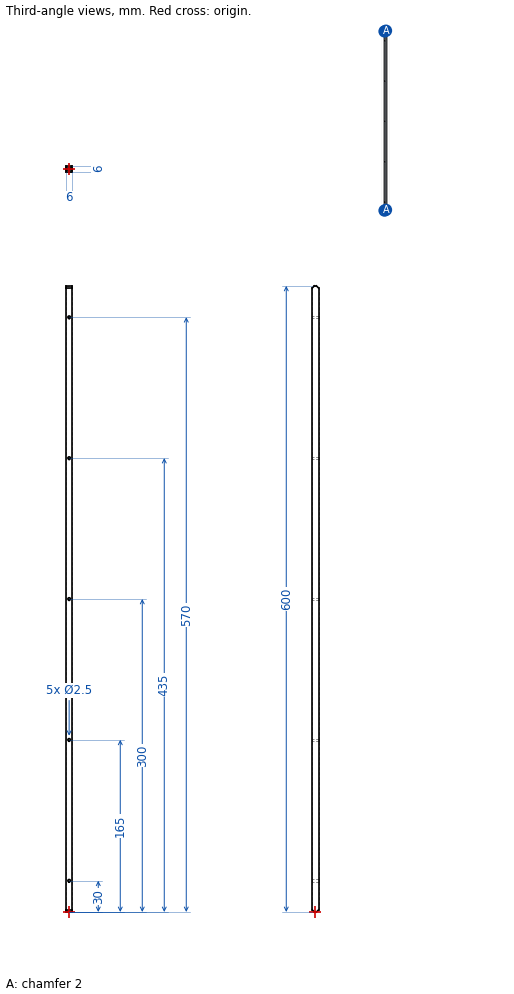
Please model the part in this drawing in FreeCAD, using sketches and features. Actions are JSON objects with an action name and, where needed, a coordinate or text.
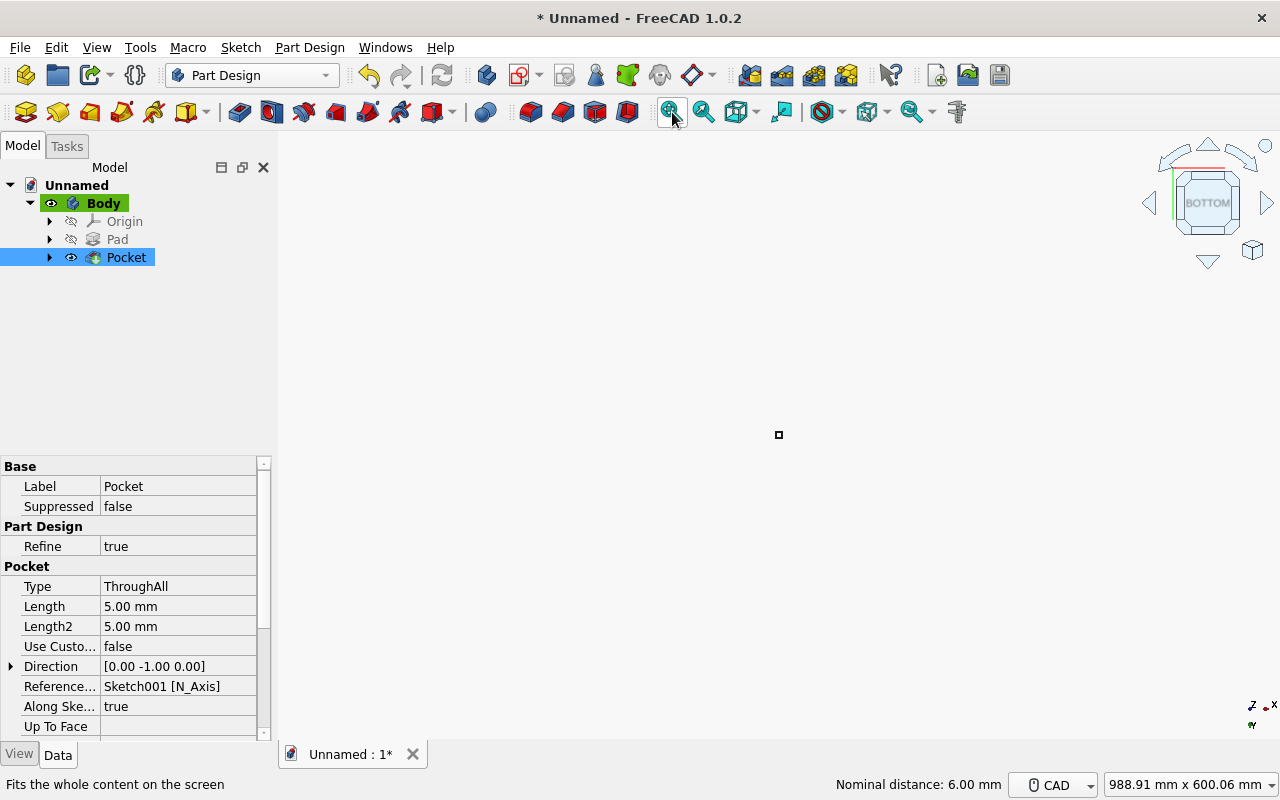
{"action": "scroll", "coordinate": [779, 431], "scroll_direction": "up", "scroll_amount": 10}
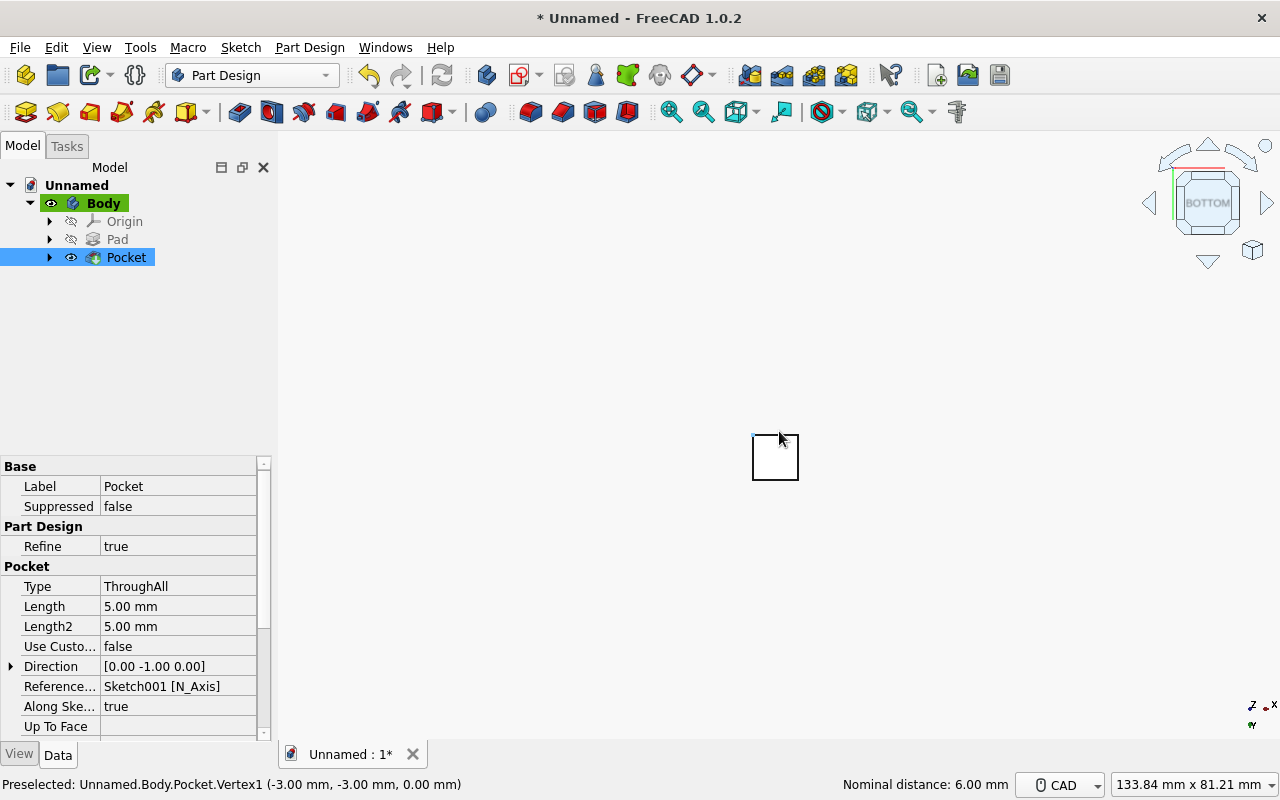
{"action": "left_click", "coordinate": [776, 434], "text": "ctrl"}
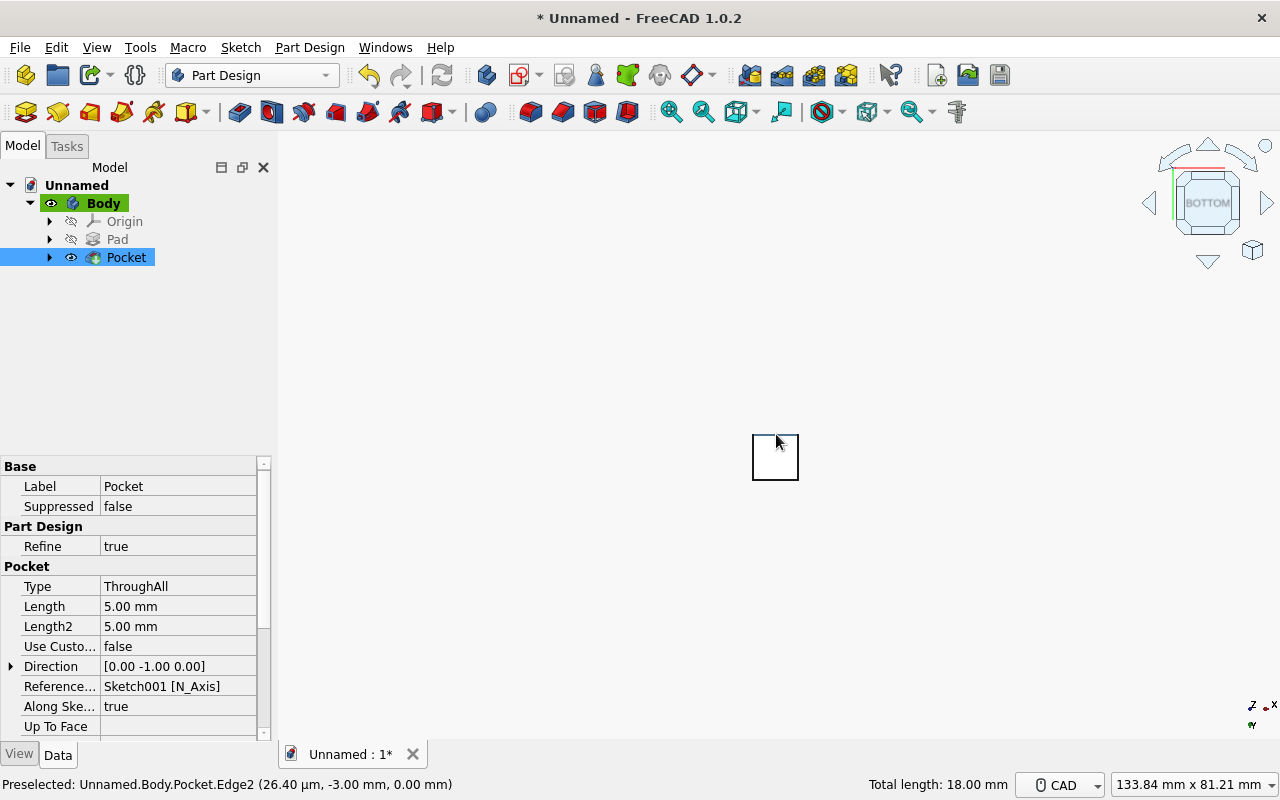
{"action": "left_click", "coordinate": [776, 479], "text": "ctrl"}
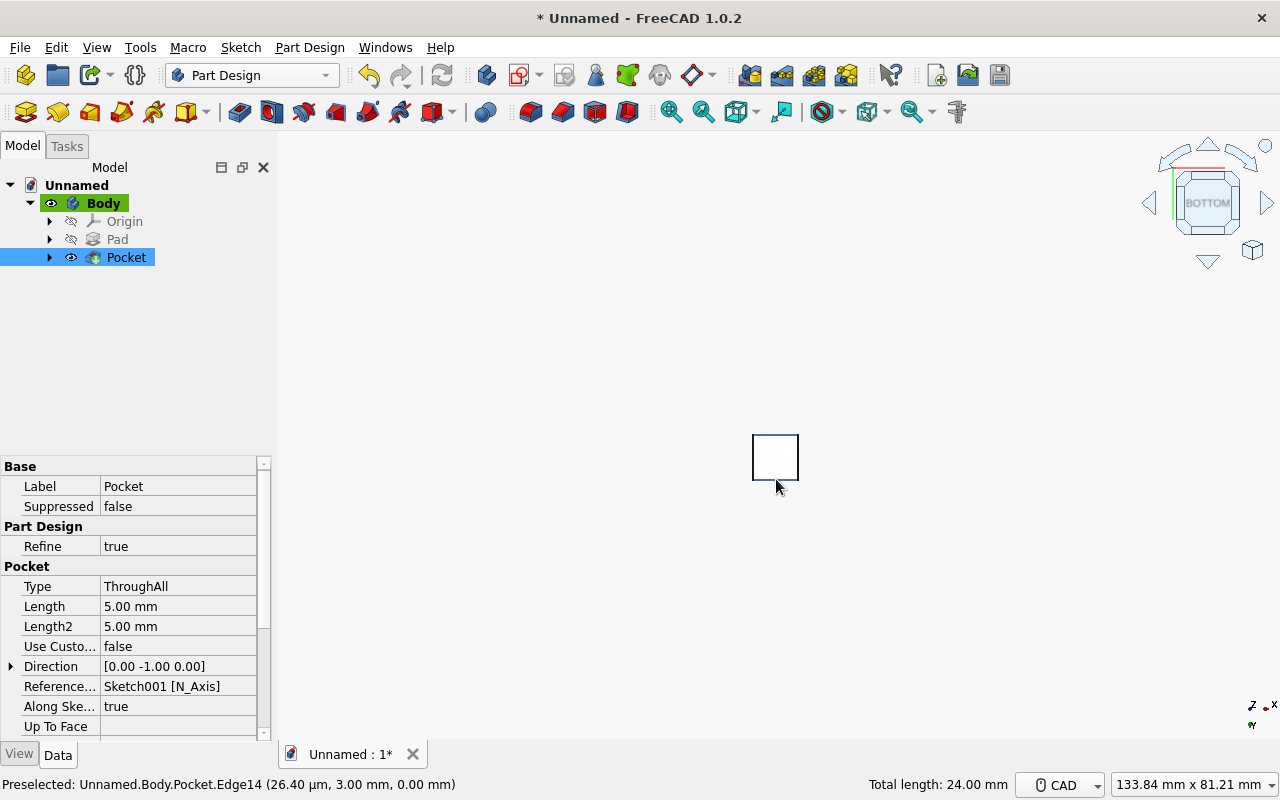
{"action": "left_click", "coordinate": [564, 112]}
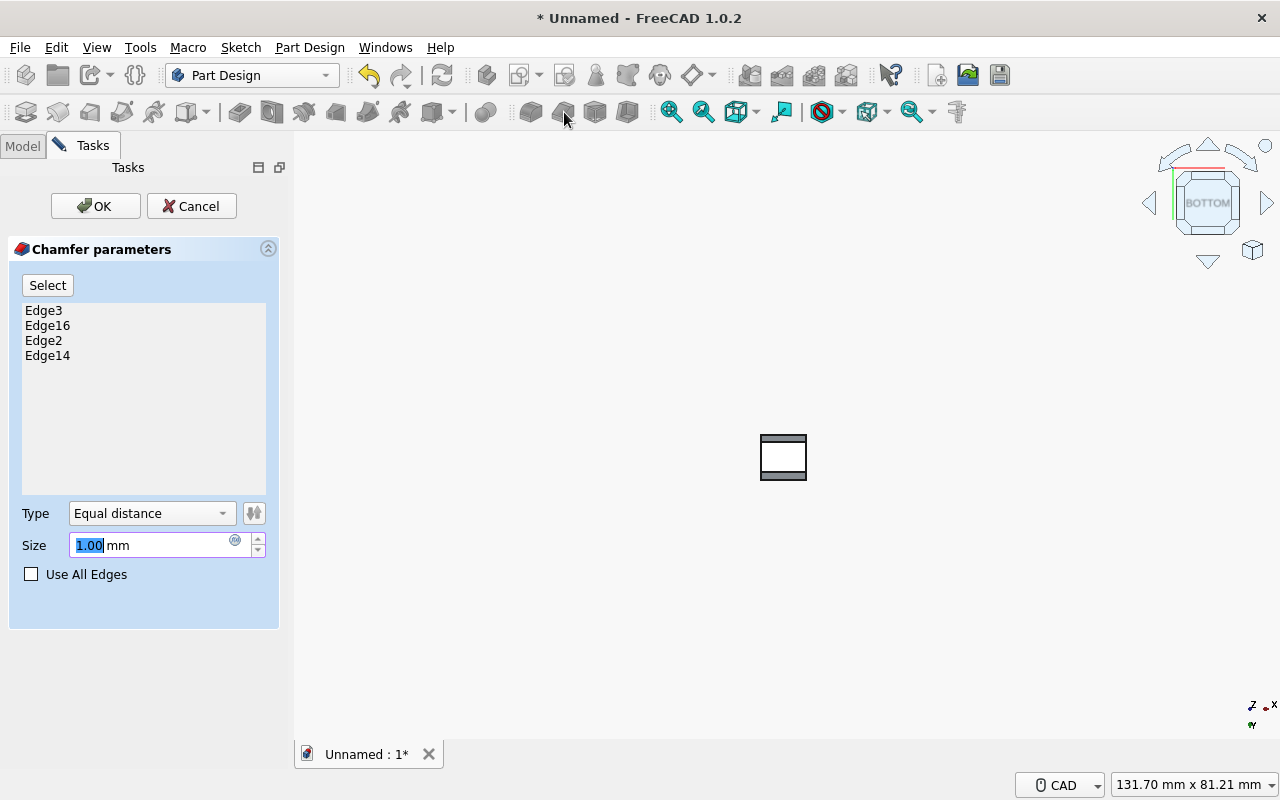
{"action": "type", "text": "2"}
{"action": "key", "text": "Tab"}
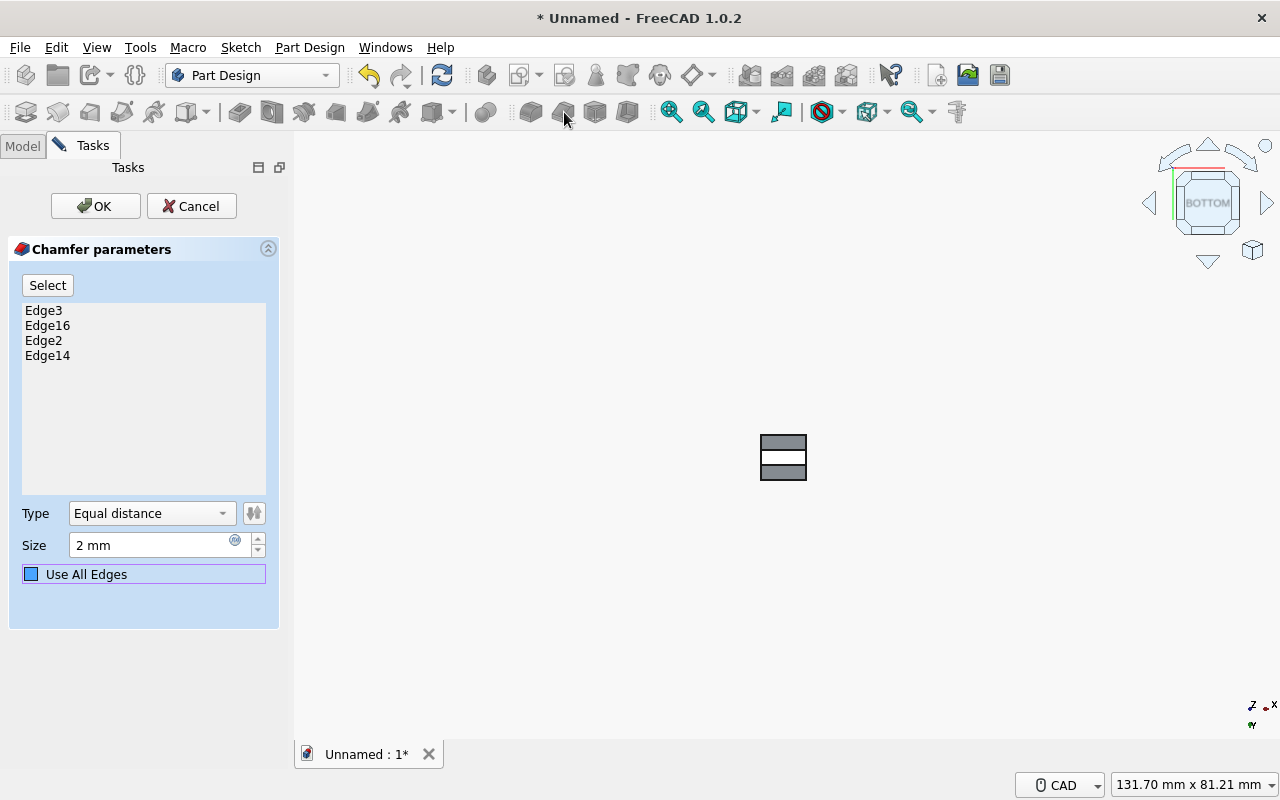
{"action": "left_click", "coordinate": [96, 206]}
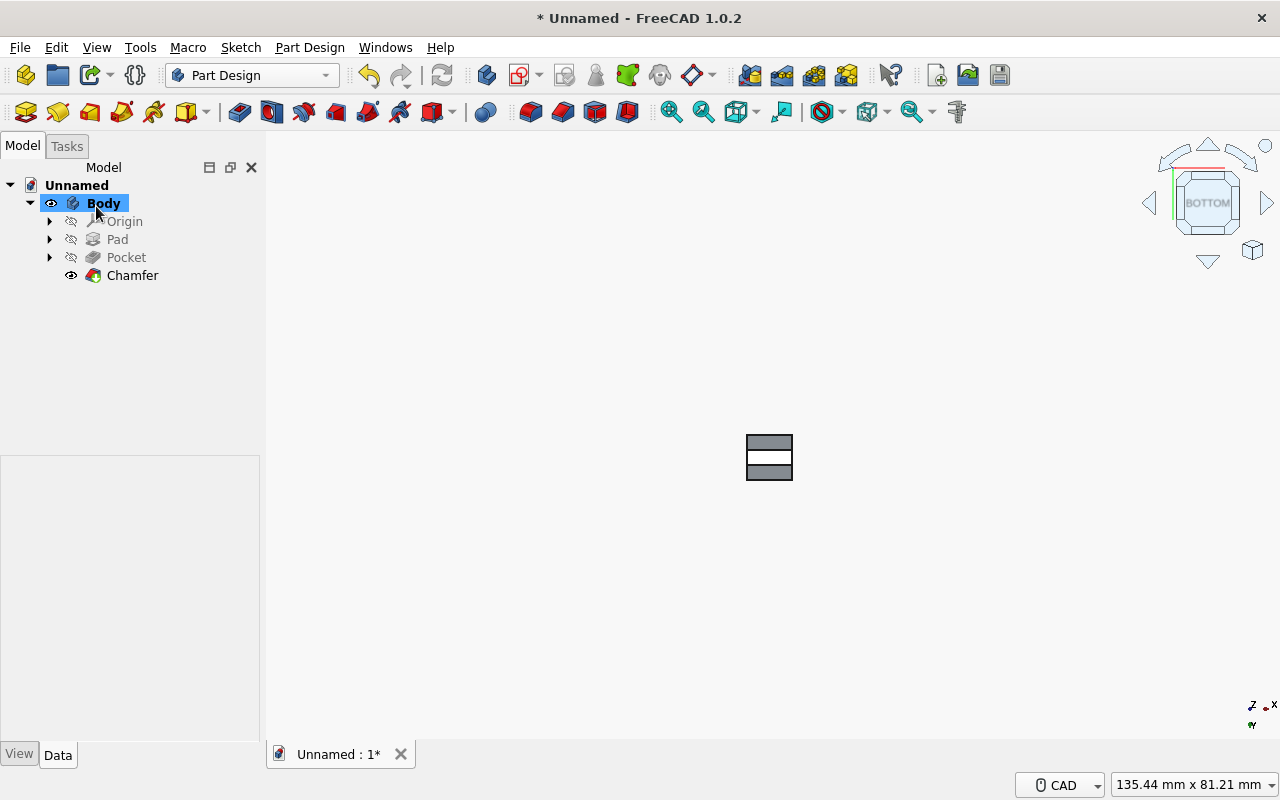
{"action": "key", "text": "0"}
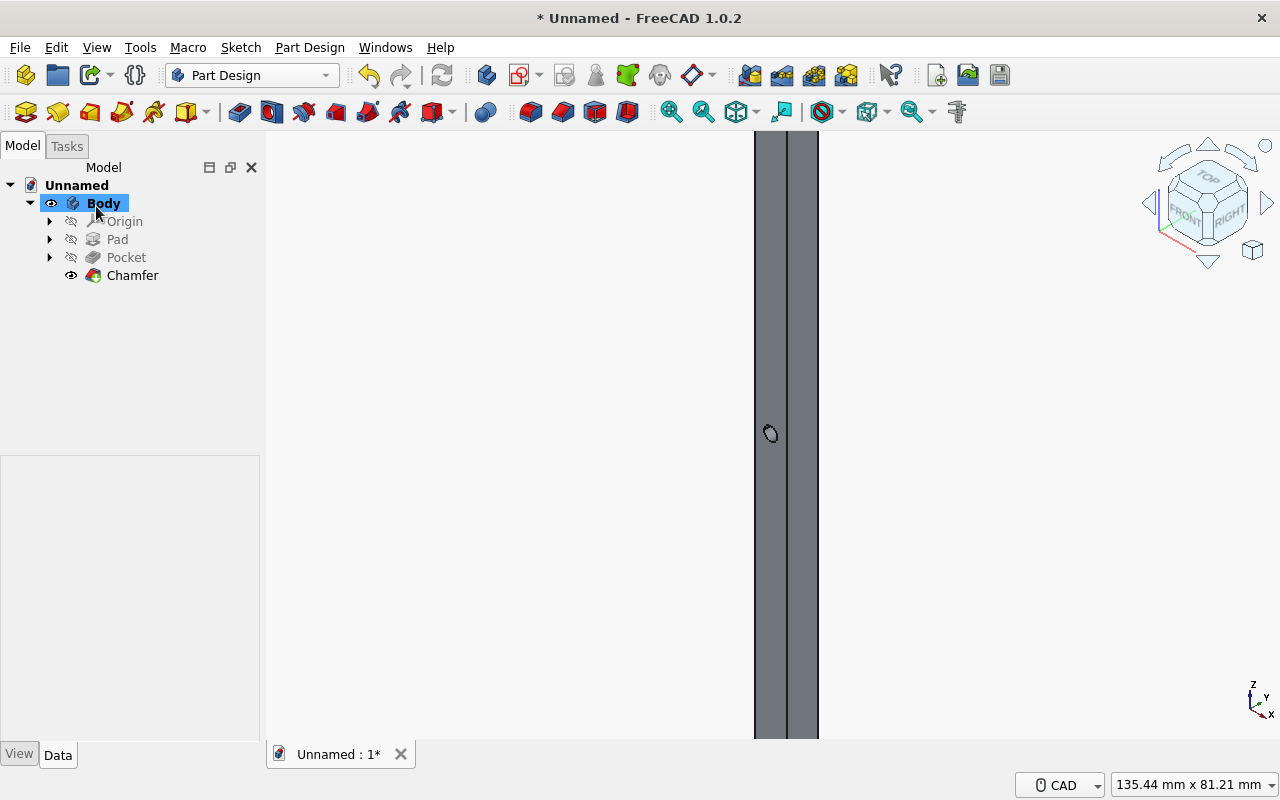
{"action": "left_click", "coordinate": [672, 112]}